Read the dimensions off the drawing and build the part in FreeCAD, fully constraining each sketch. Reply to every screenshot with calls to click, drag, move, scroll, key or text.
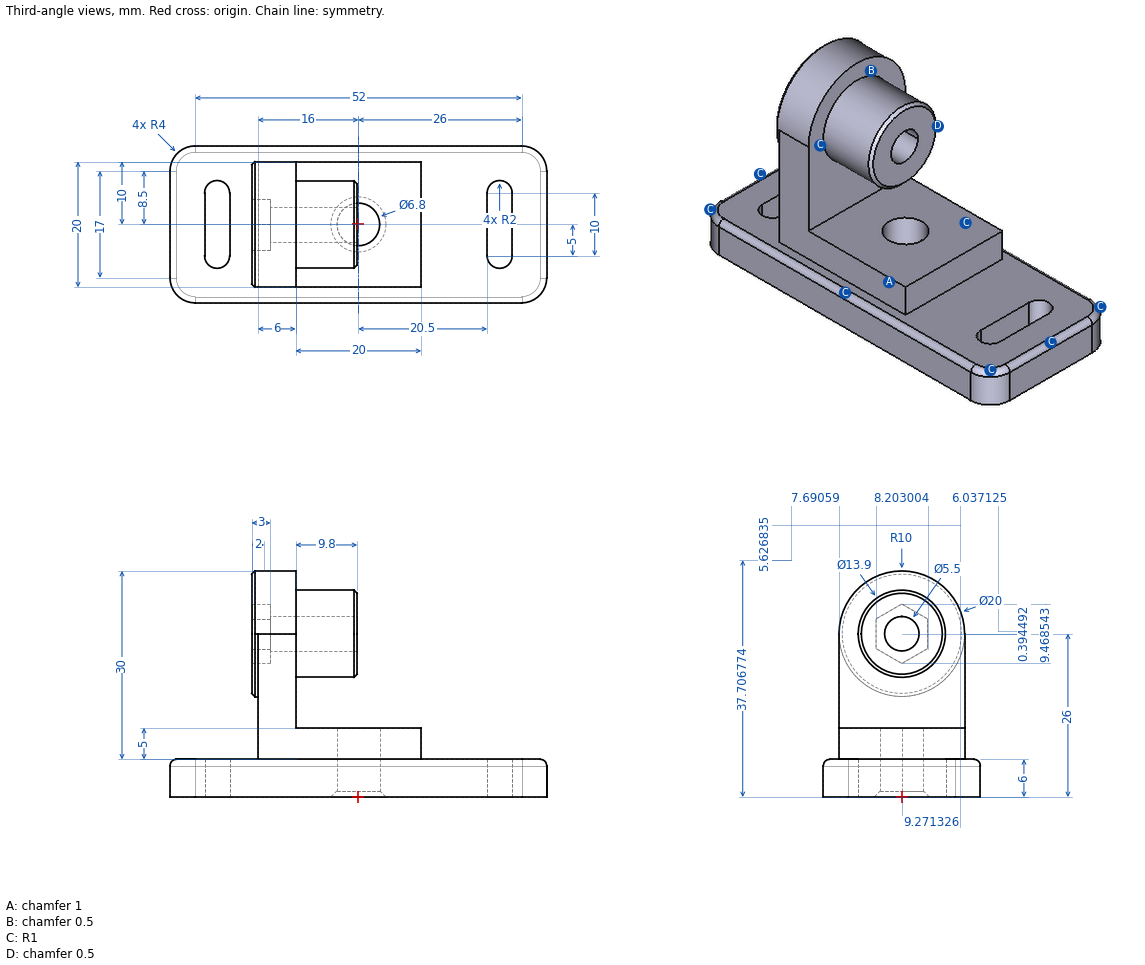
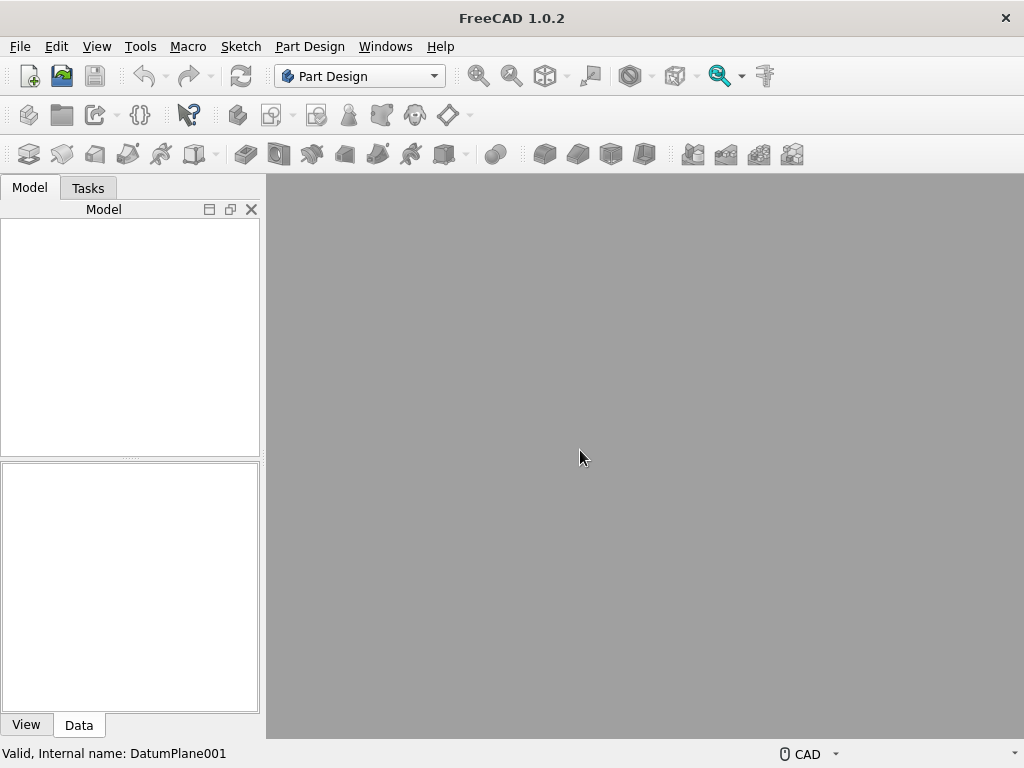
key(ctrl+n)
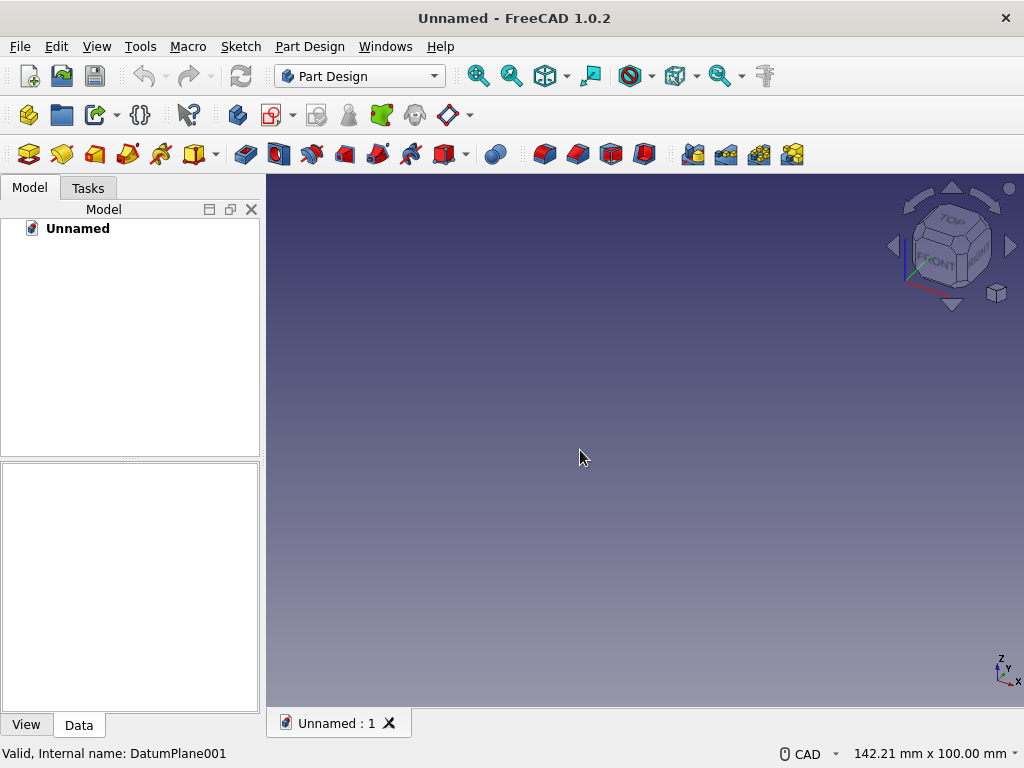
click(270, 116)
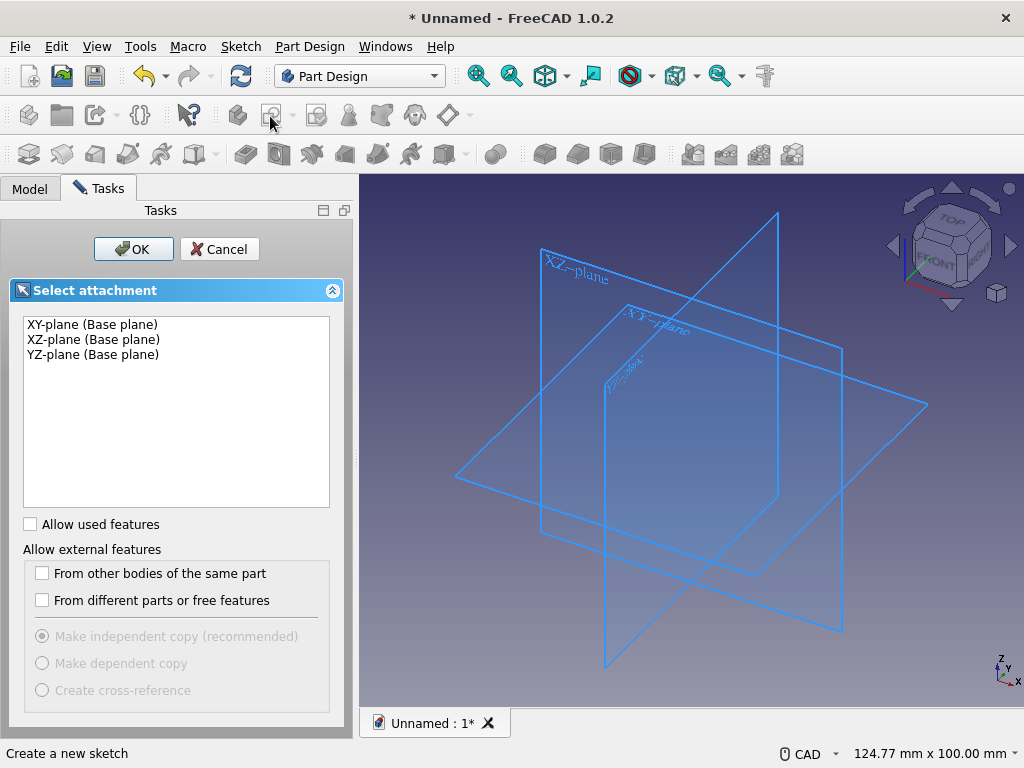
click(84, 324)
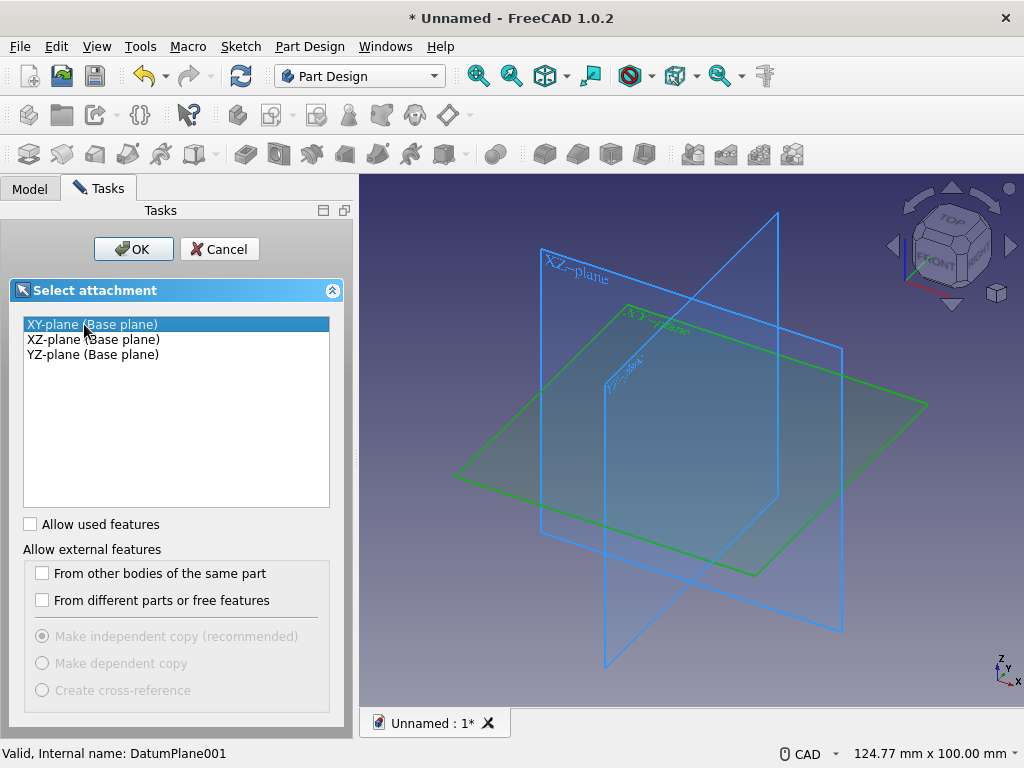
click(134, 249)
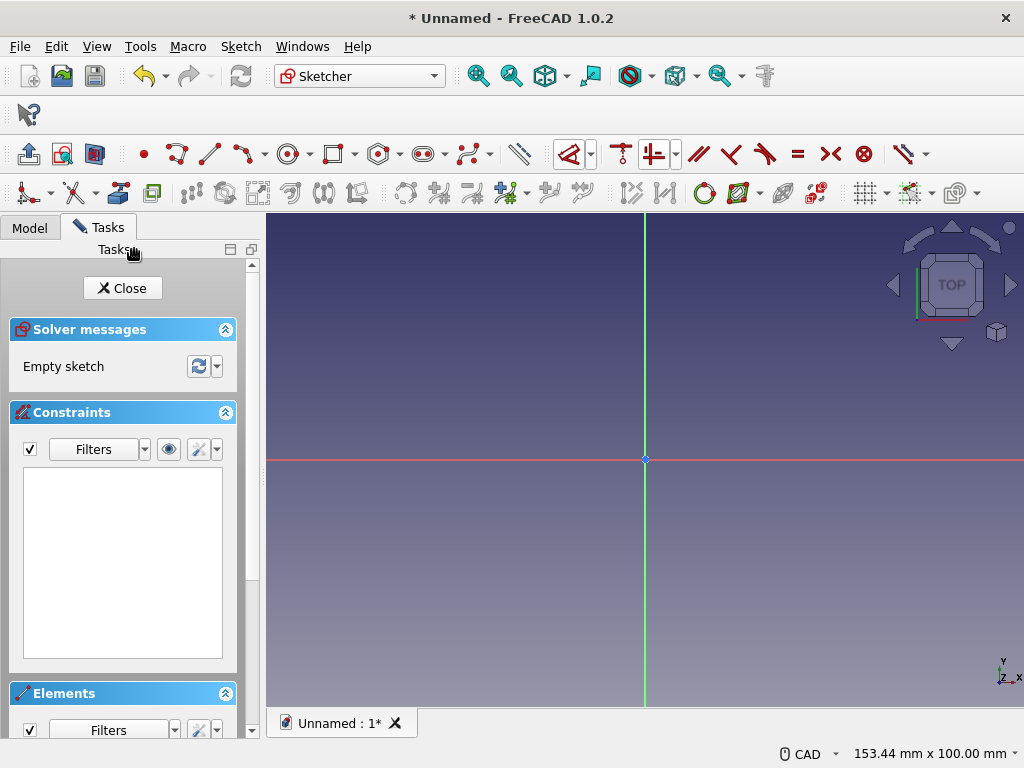
click(210, 154)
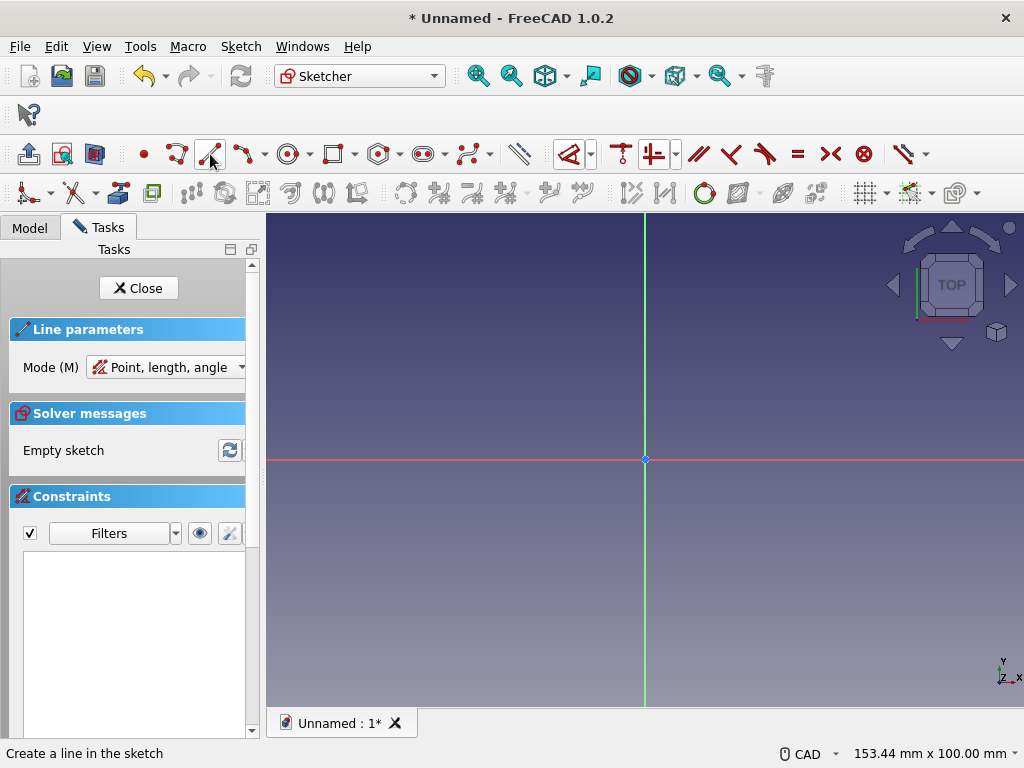
click(773, 398)
click(517, 398)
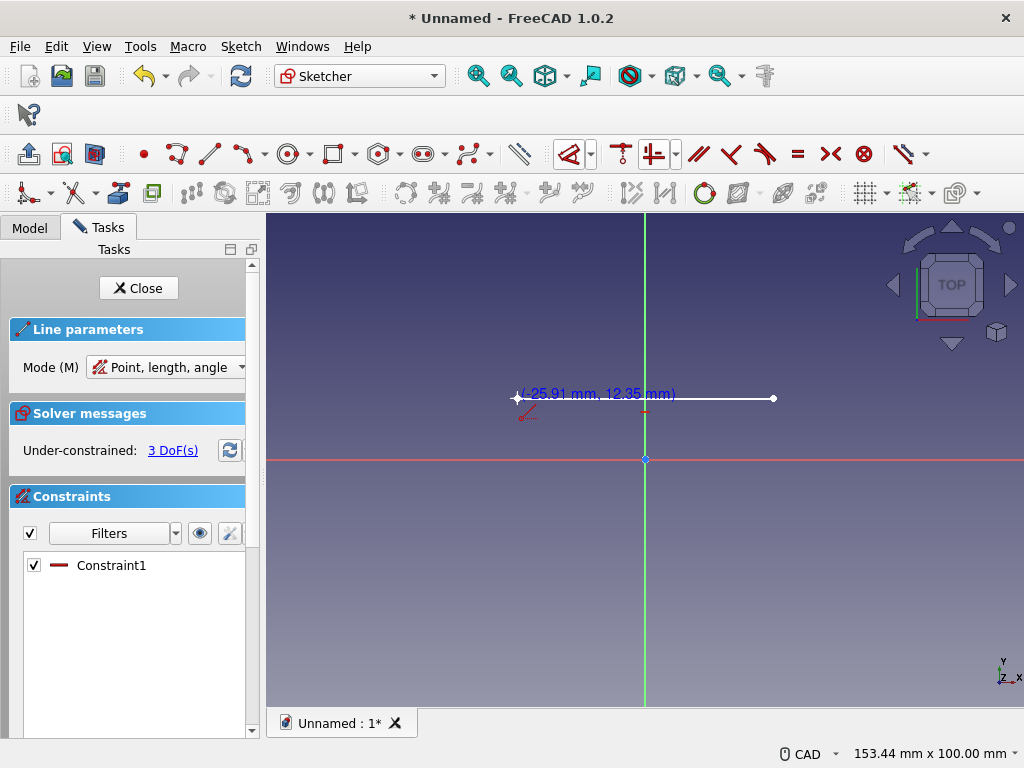
click(497, 418)
click(497, 502)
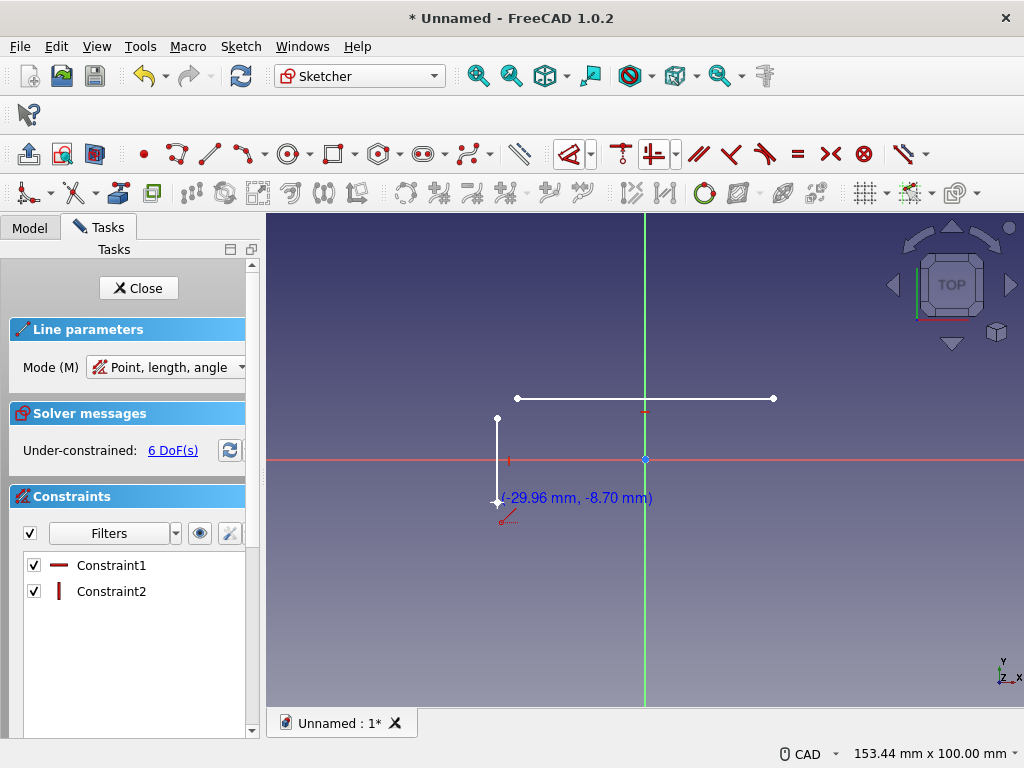
click(517, 522)
click(773, 522)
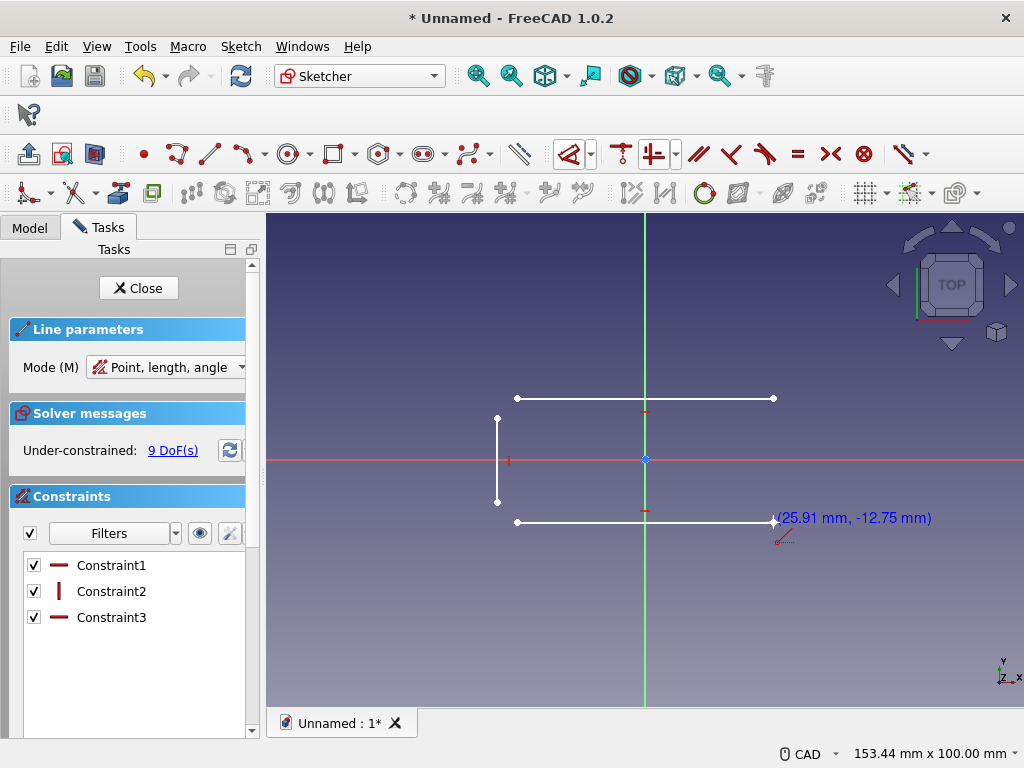
click(793, 502)
click(793, 418)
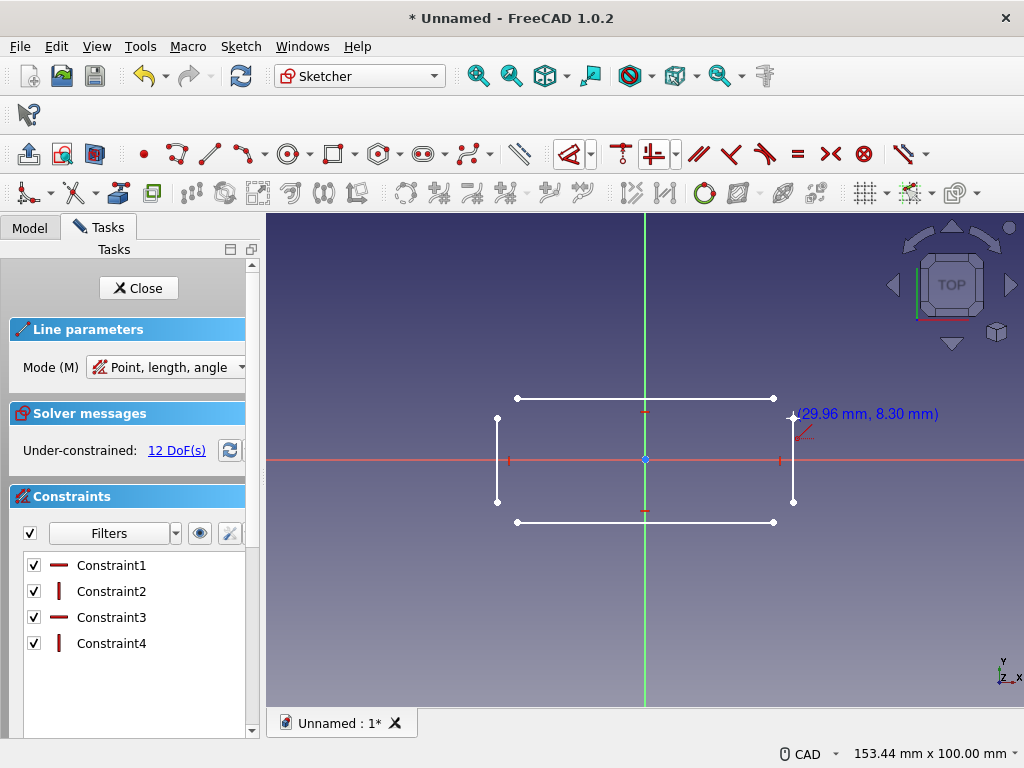
key(g)
key(3)
key(a)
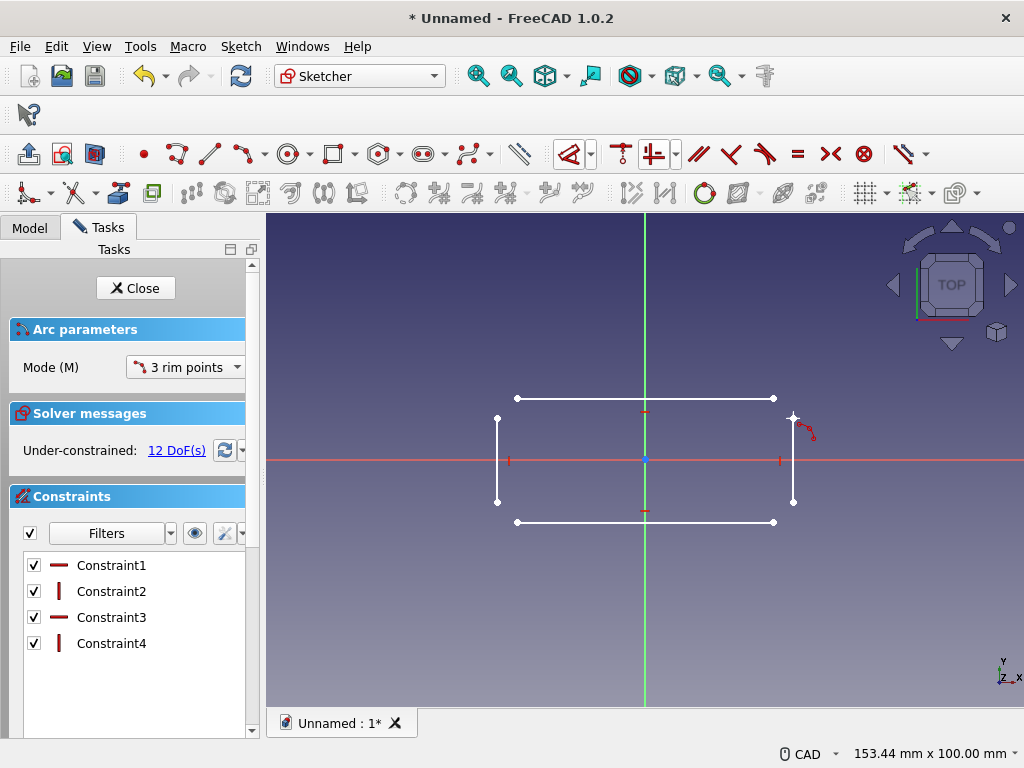
click(517, 399)
click(497, 419)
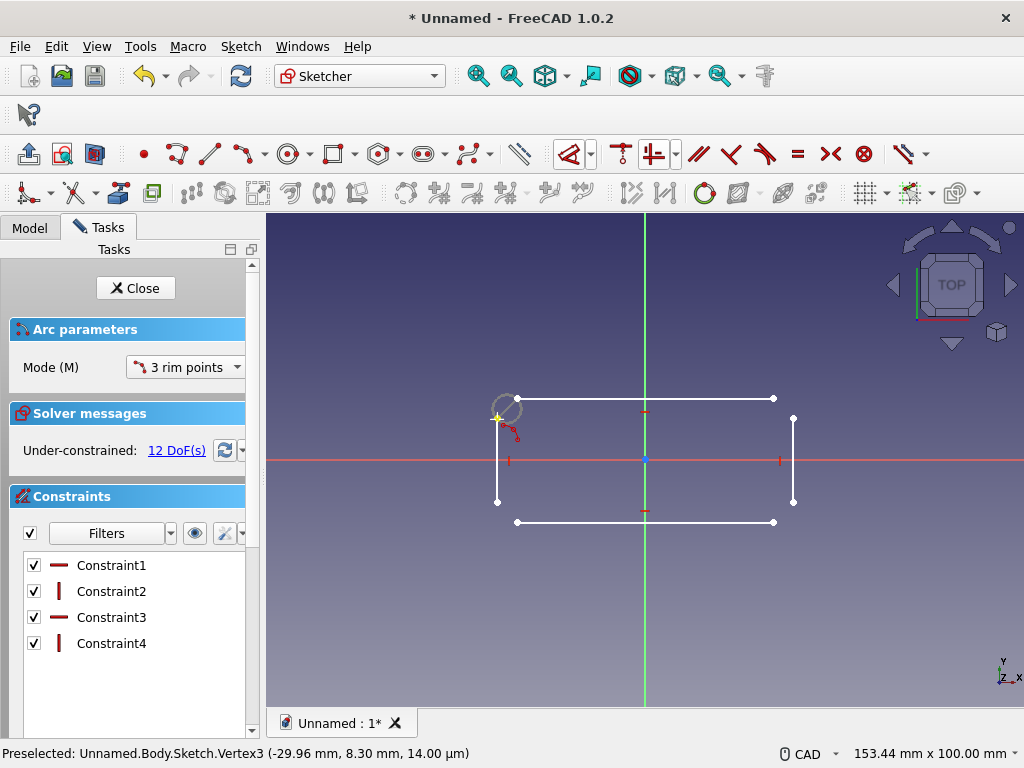
scroll(503, 404, up, 6)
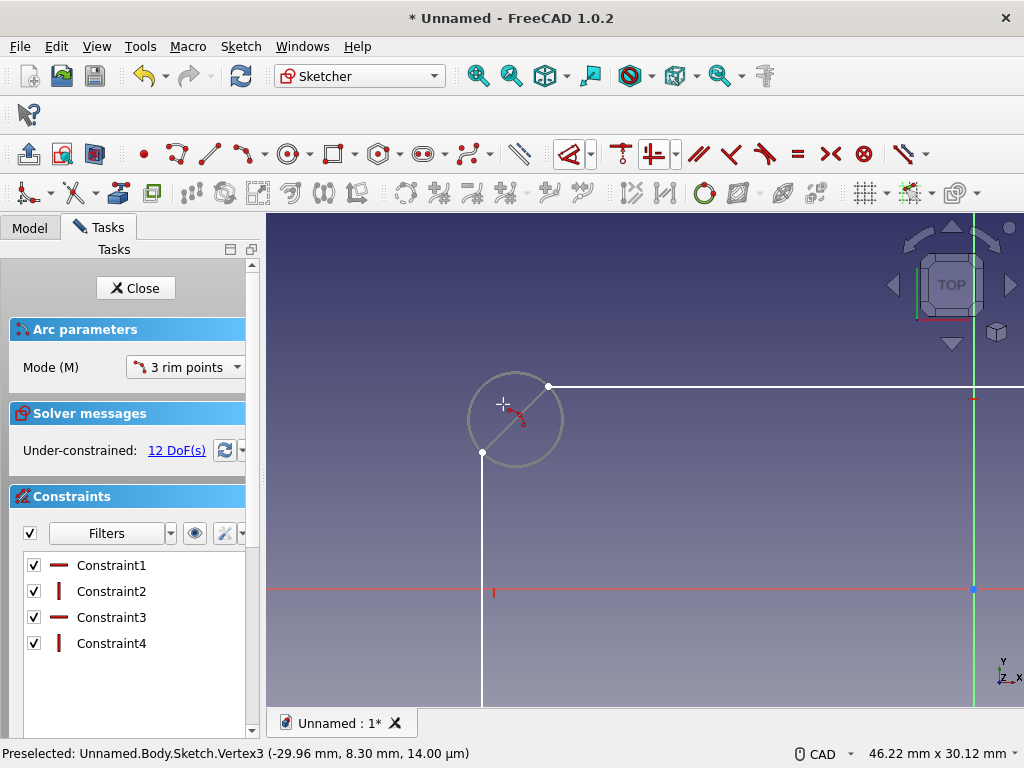
click(501, 403)